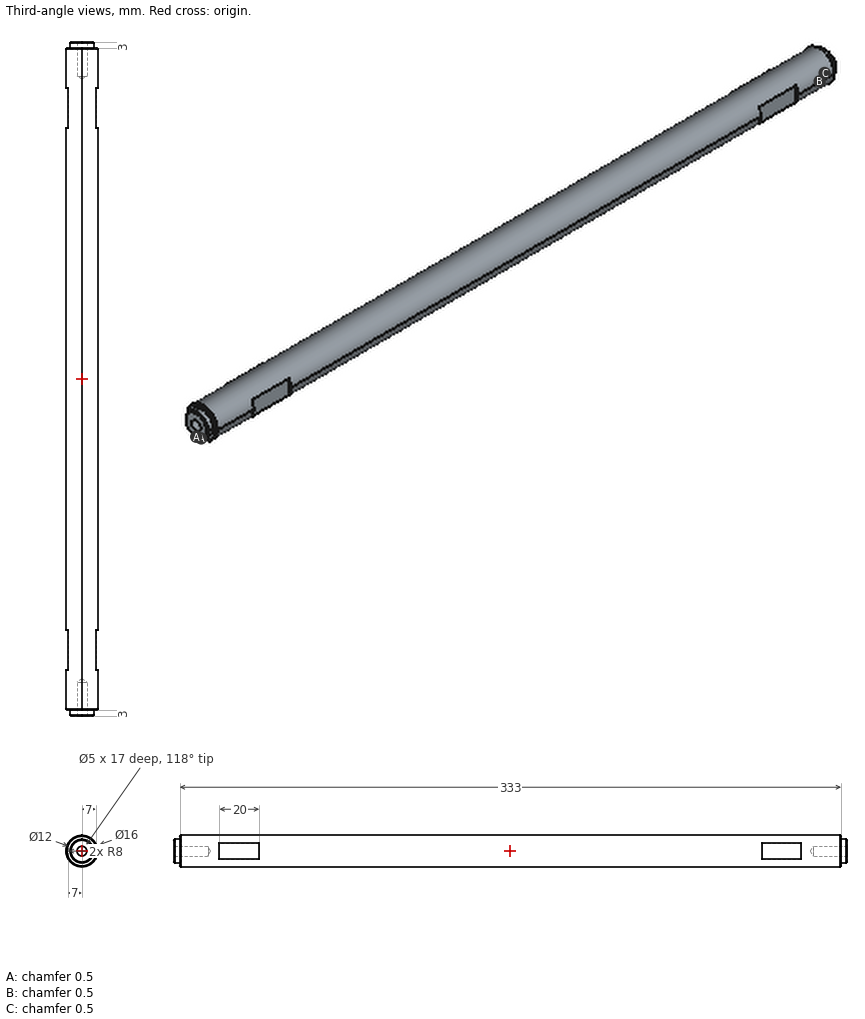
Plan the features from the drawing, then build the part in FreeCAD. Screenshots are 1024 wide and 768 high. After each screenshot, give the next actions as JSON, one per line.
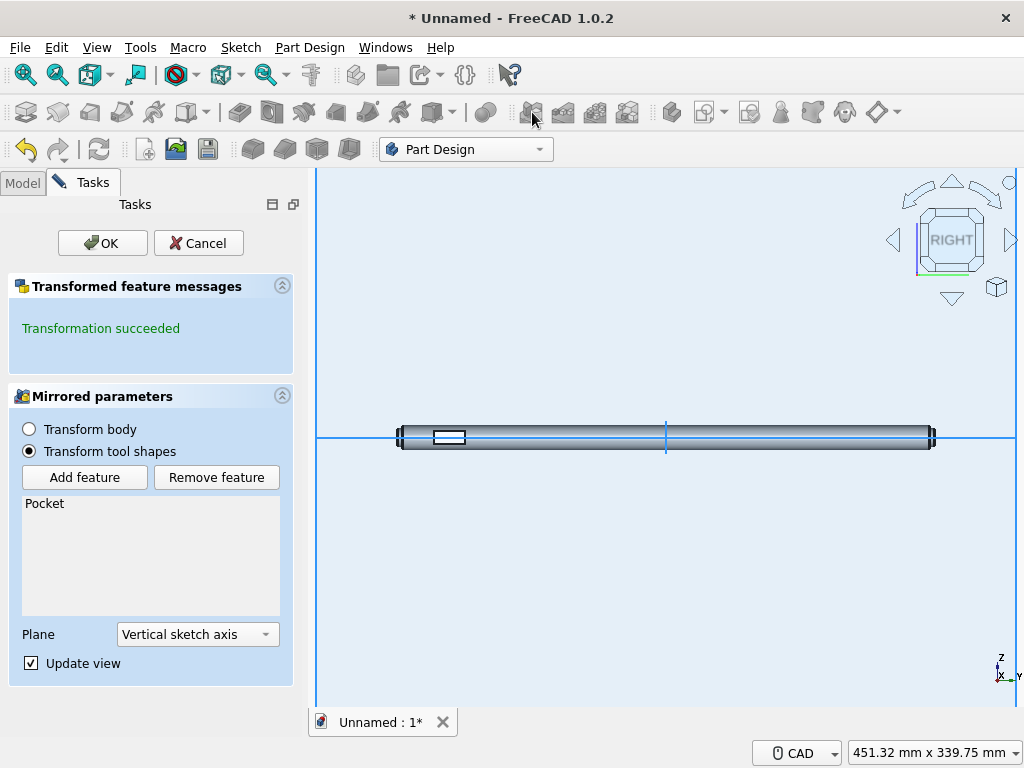
{"action": "left_click", "coordinate": [198, 634]}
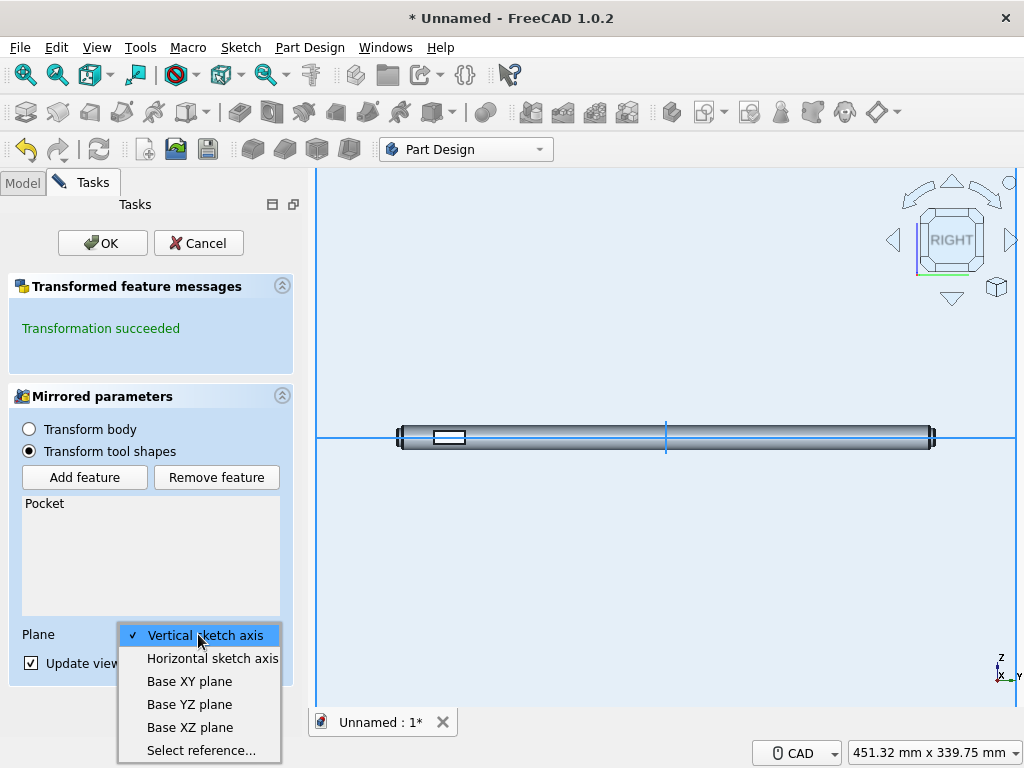
{"action": "left_click", "coordinate": [198, 728]}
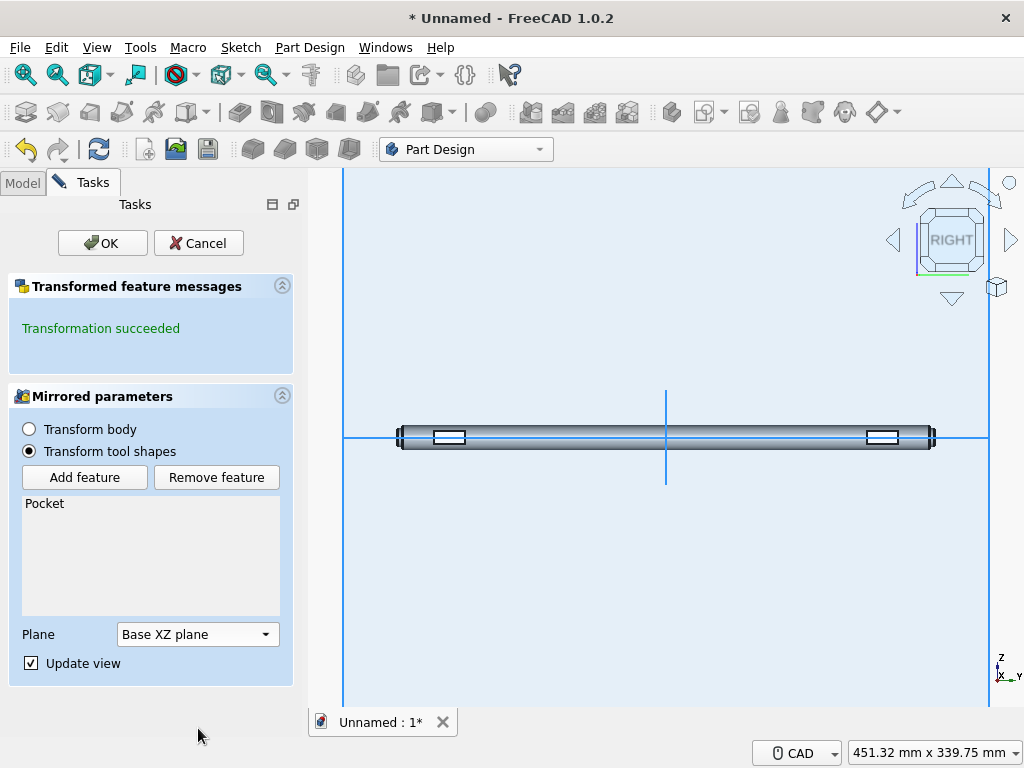
{"action": "left_click", "coordinate": [103, 243]}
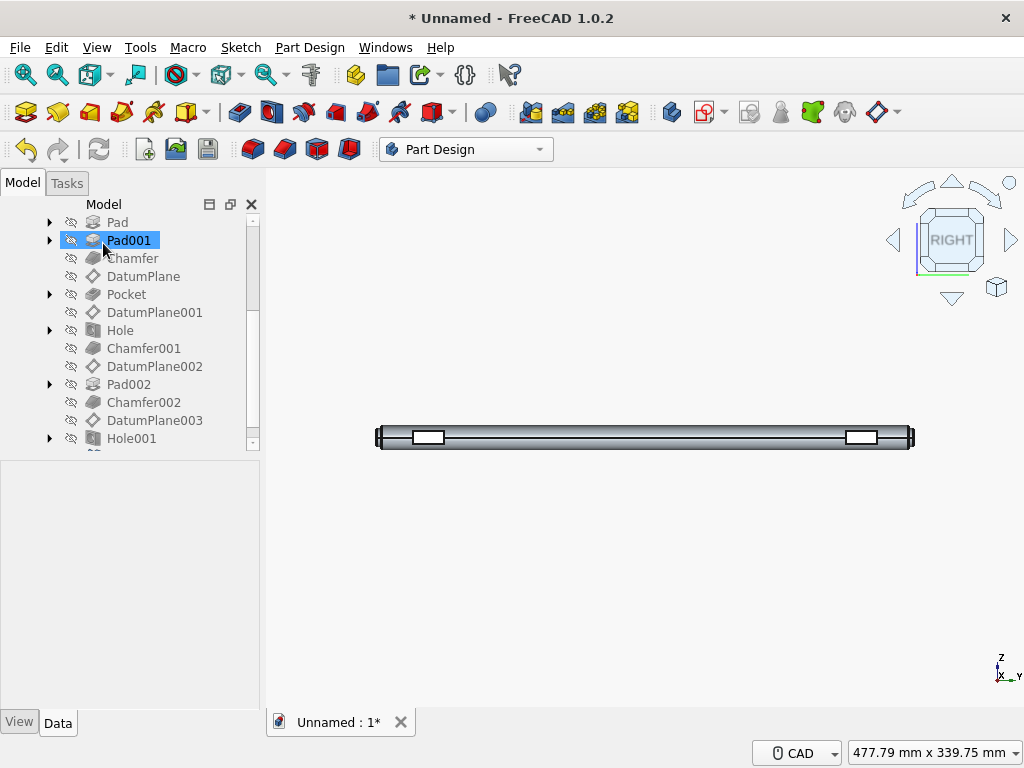
{"action": "key", "text": "0"}